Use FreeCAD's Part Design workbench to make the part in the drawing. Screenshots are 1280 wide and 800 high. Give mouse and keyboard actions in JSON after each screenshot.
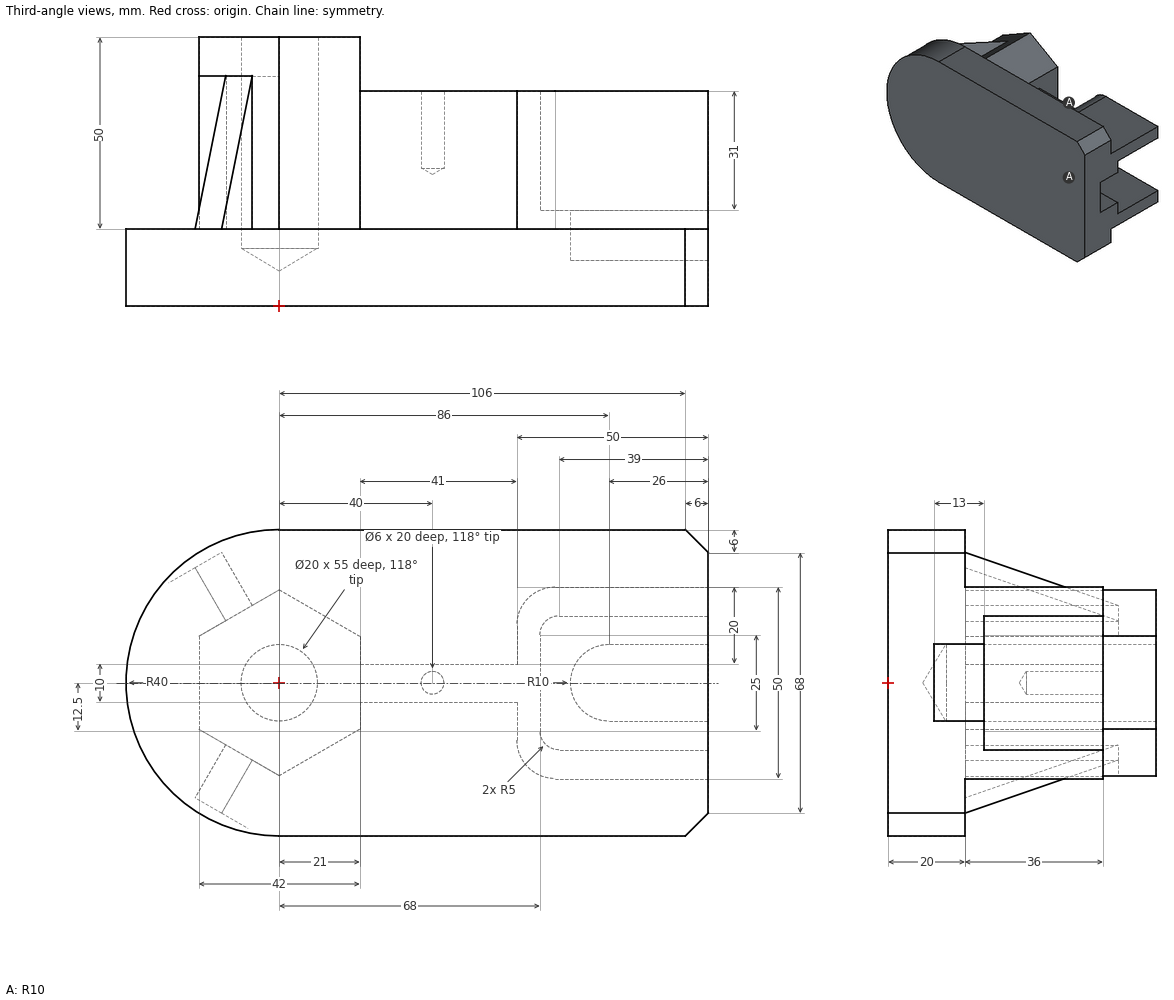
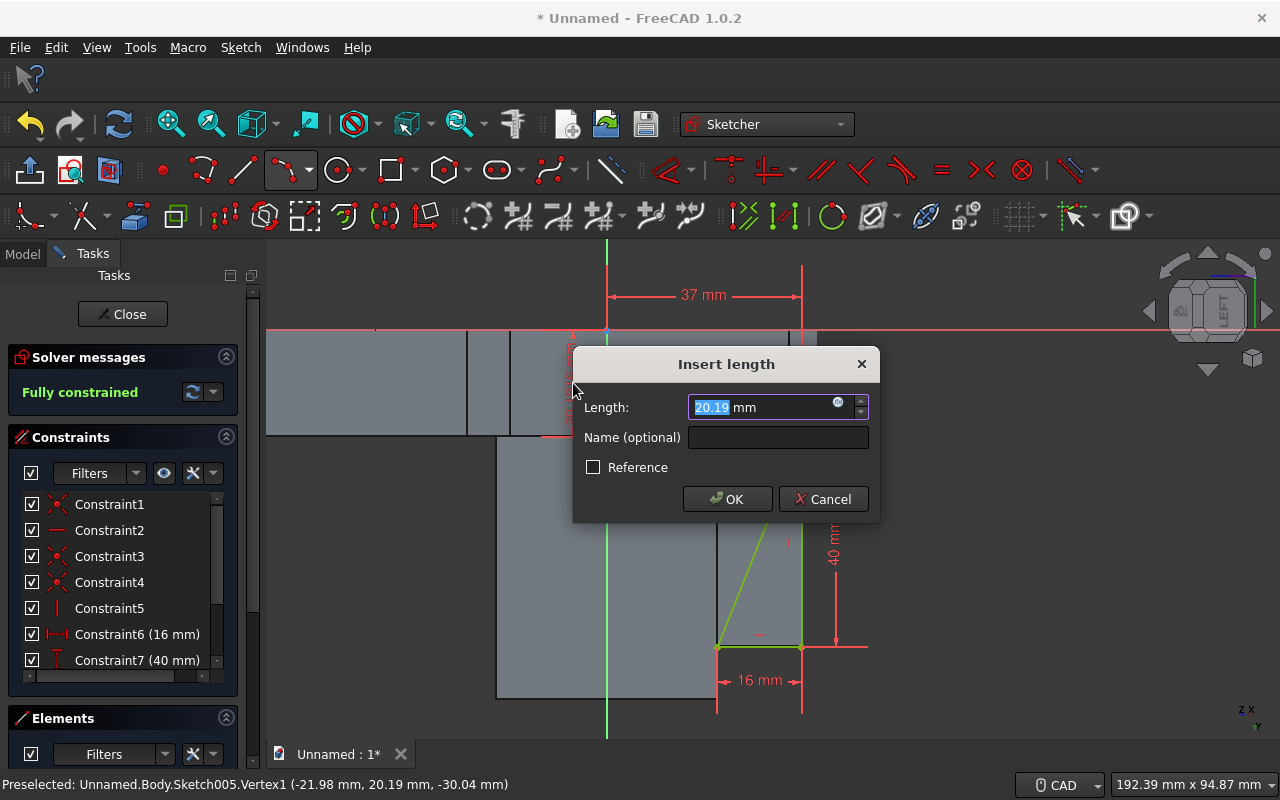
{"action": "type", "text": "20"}
{"action": "key", "text": "Return"}
{"action": "key", "text": "Escape"}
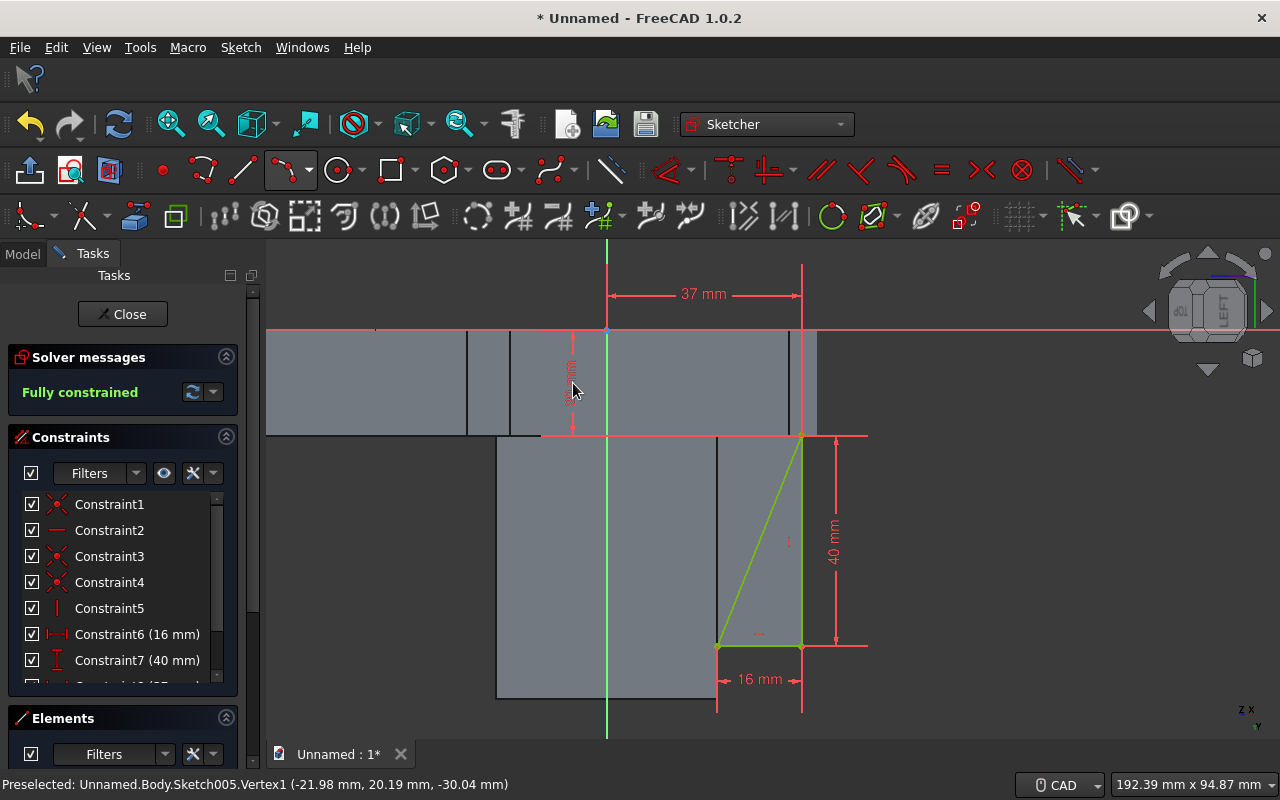
{"action": "left_click", "coordinate": [123, 314]}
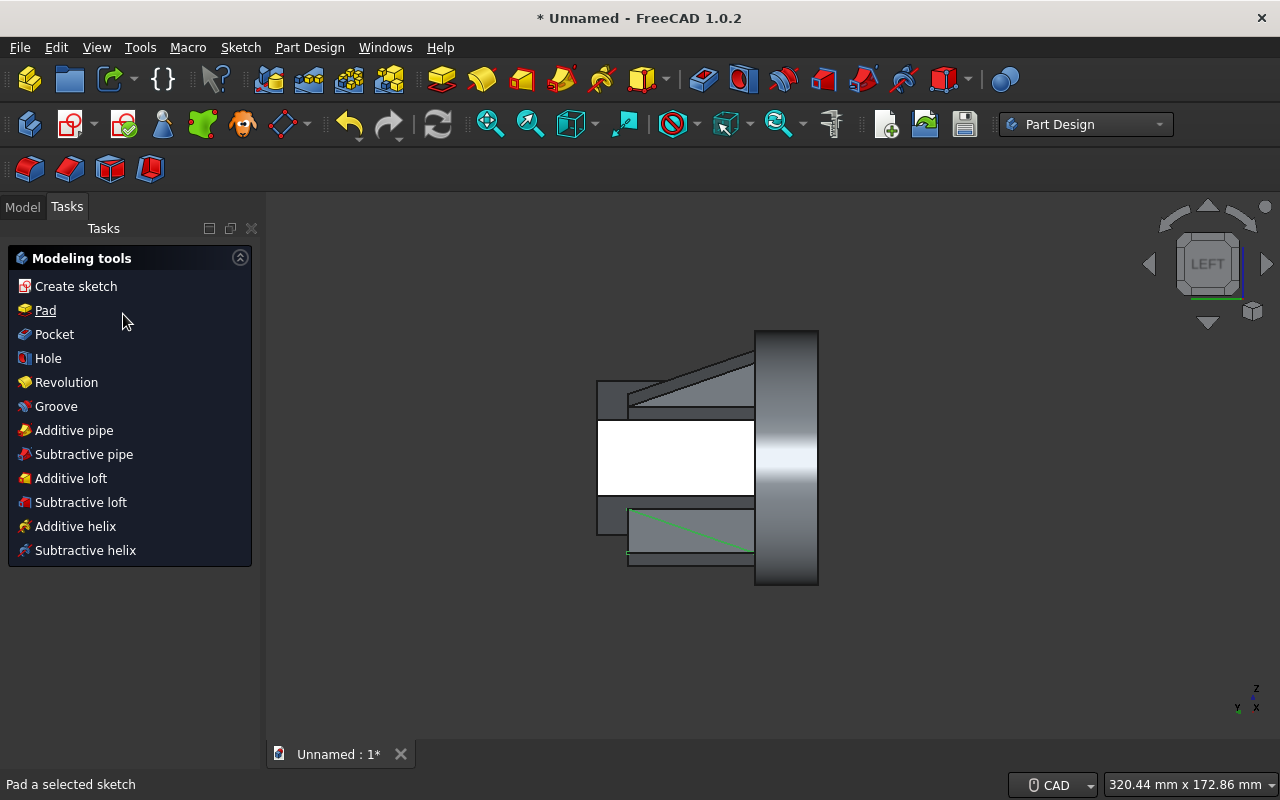
{"action": "left_click", "coordinate": [704, 80]}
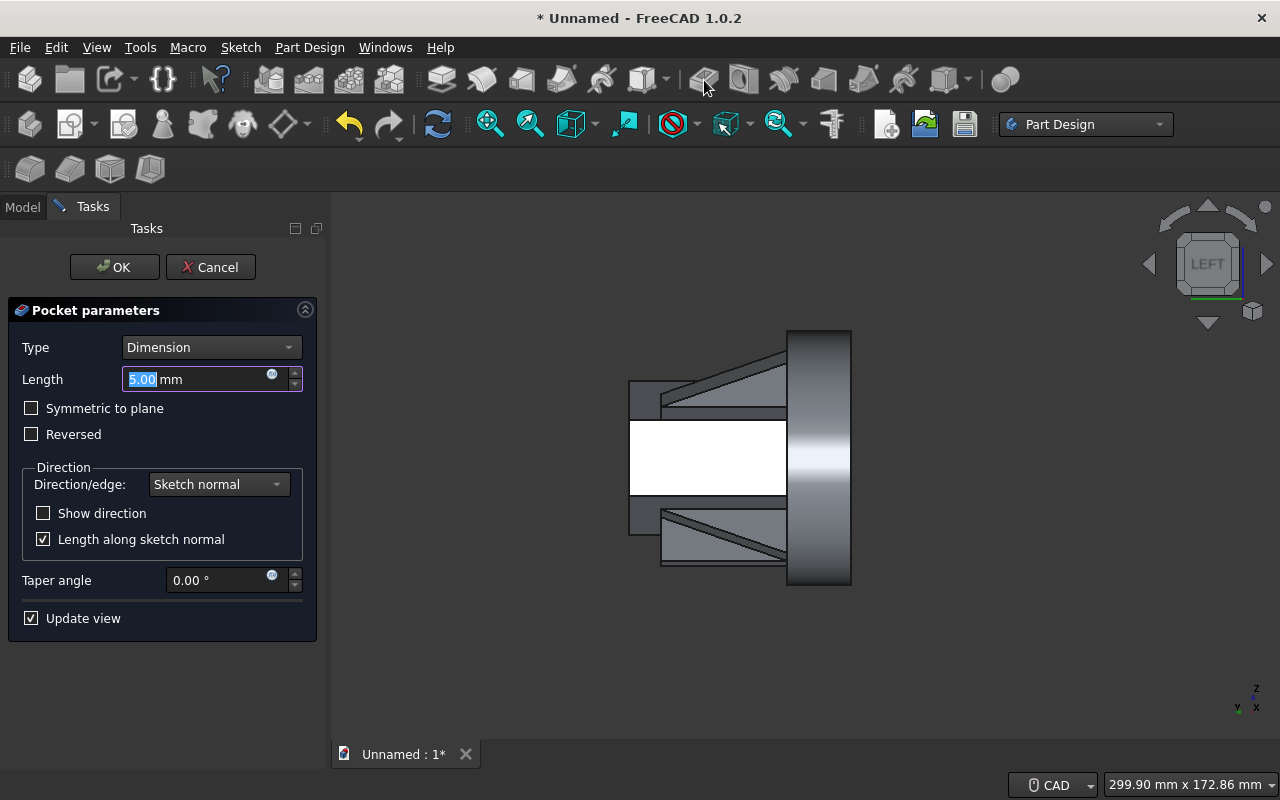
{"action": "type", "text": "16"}
{"action": "key", "text": "Tab"}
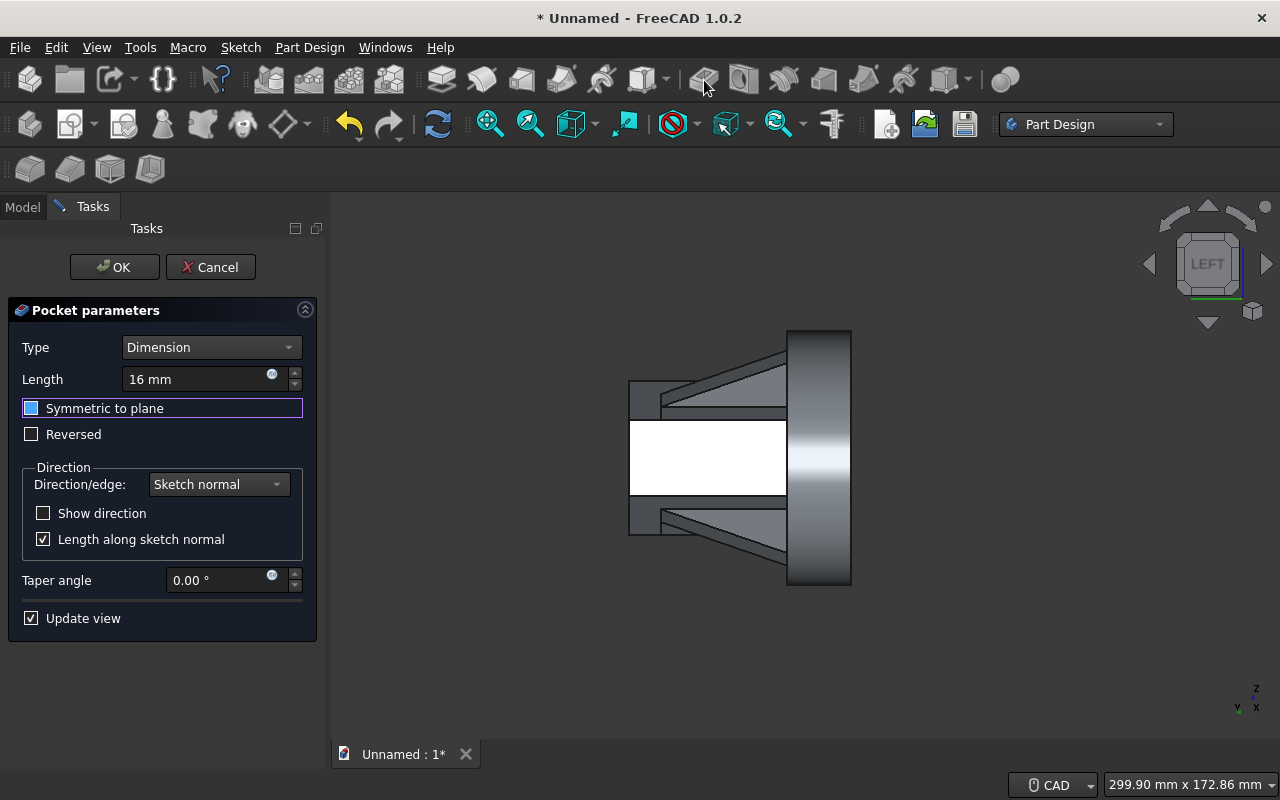
{"action": "left_click", "coordinate": [115, 267]}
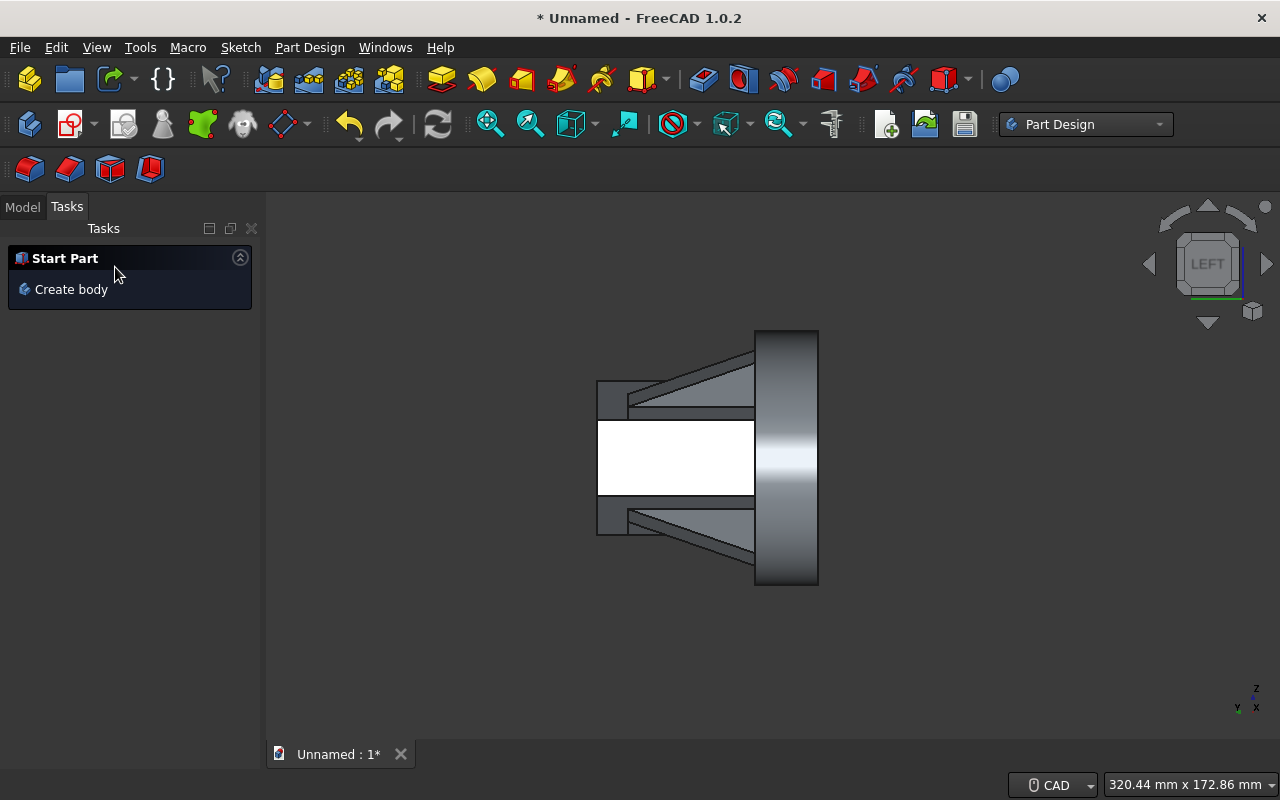
{"action": "key", "text": "4"}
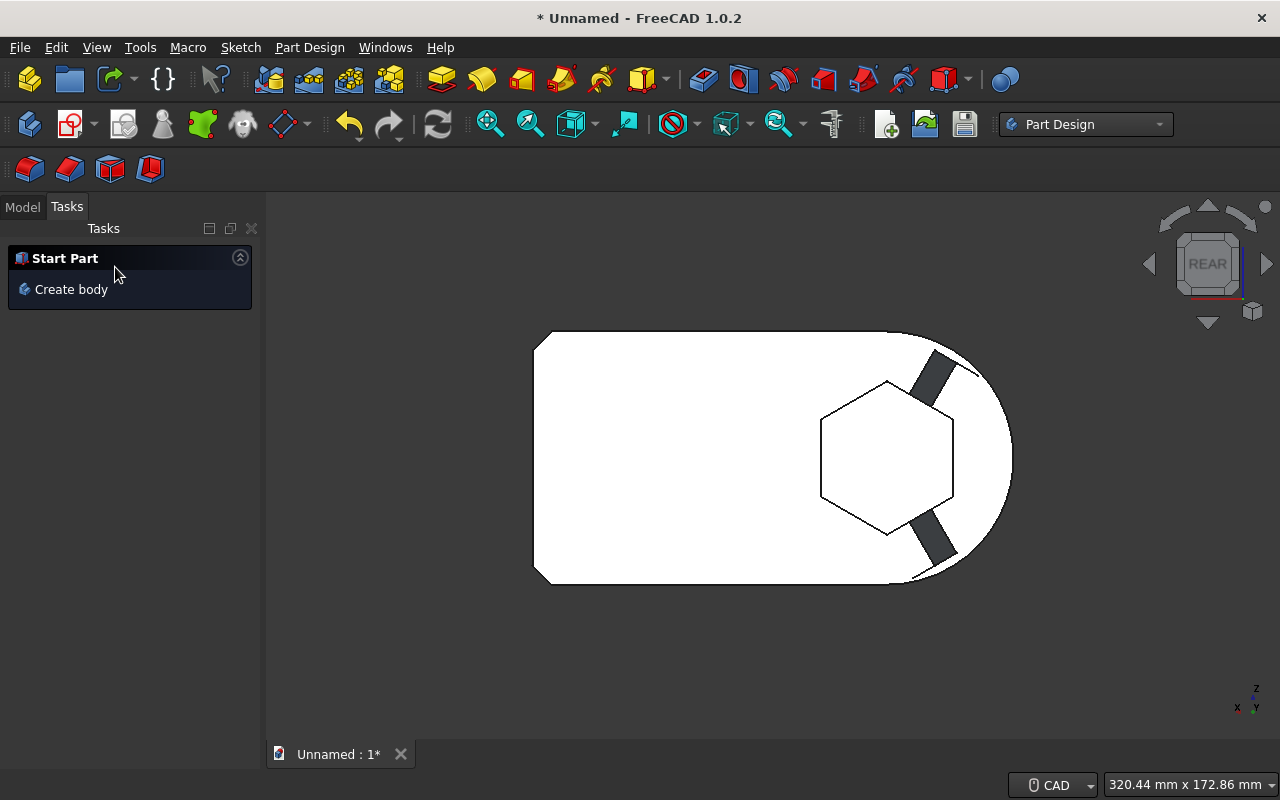
{"action": "left_click", "coordinate": [887, 457]}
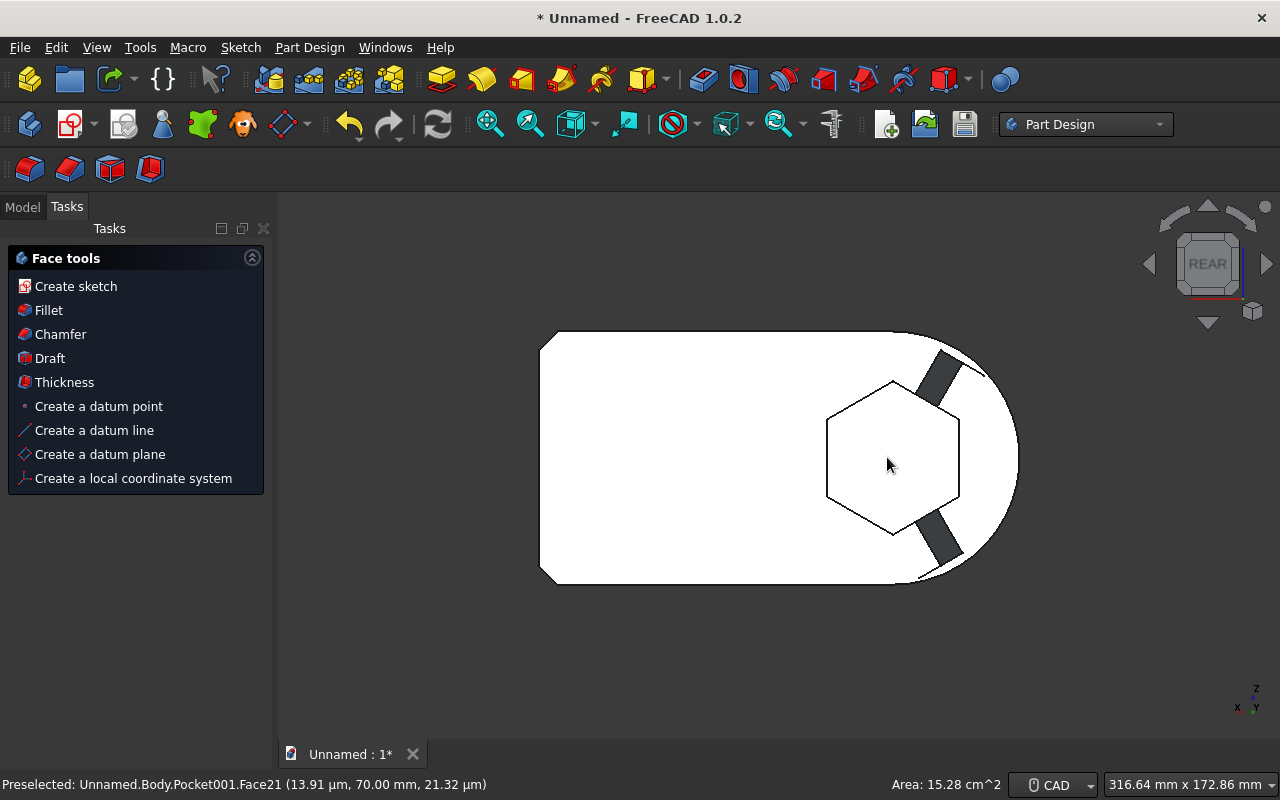
{"action": "left_click", "coordinate": [70, 124]}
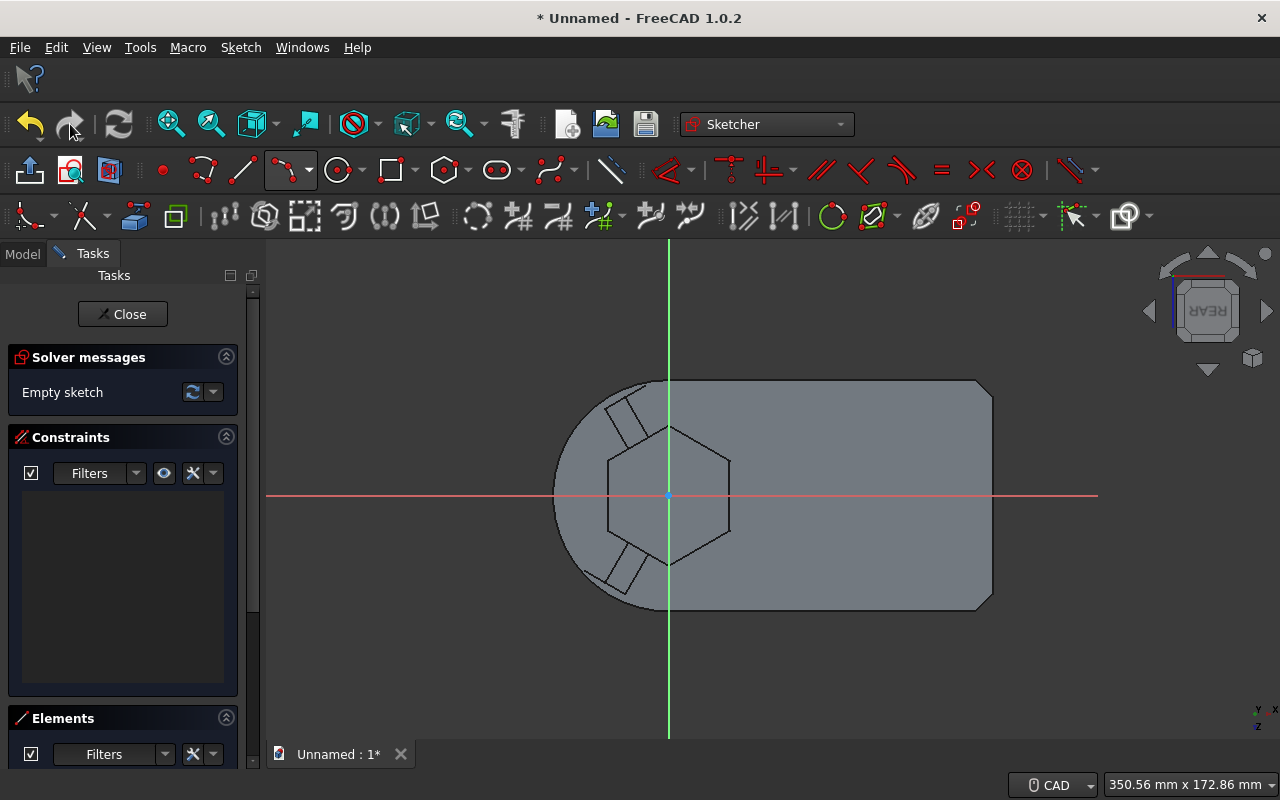
{"action": "scroll", "coordinate": [660, 498], "scroll_direction": "up", "scroll_amount": 8}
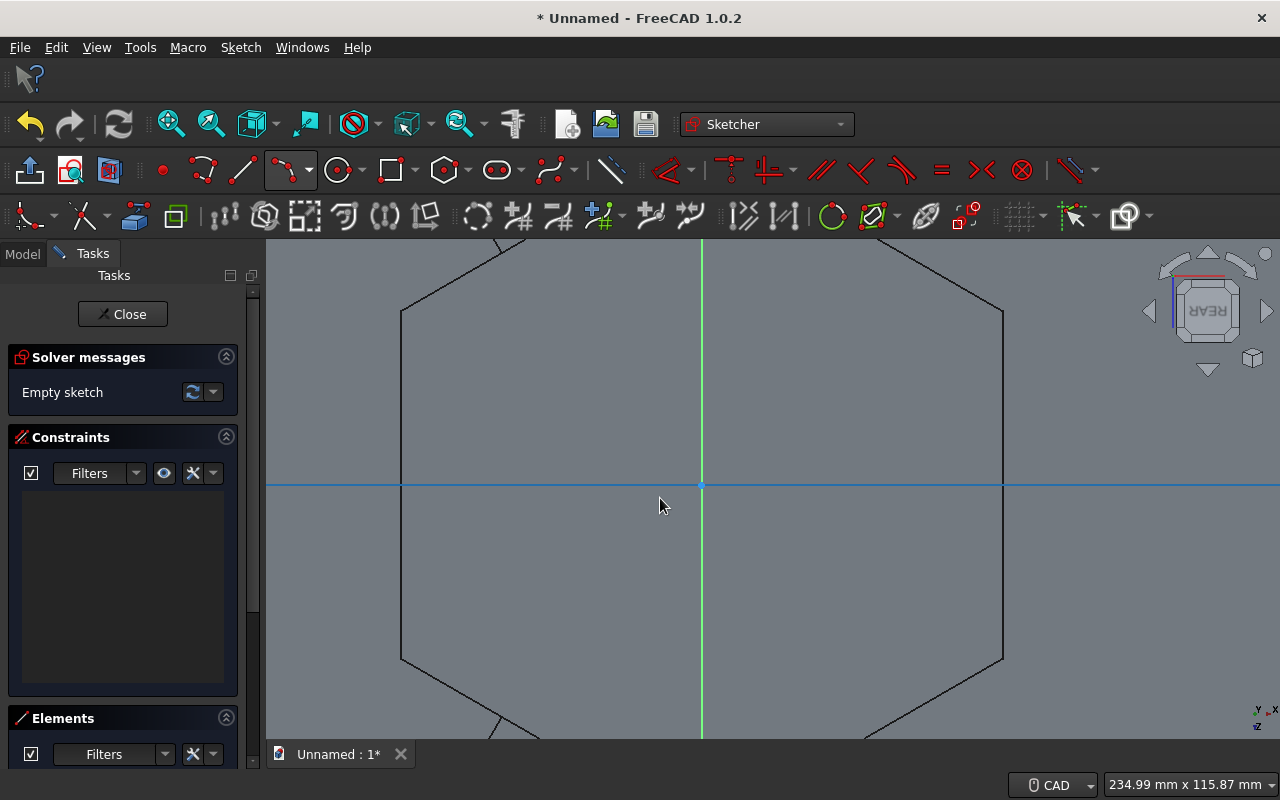
{"action": "left_click", "coordinate": [338, 170]}